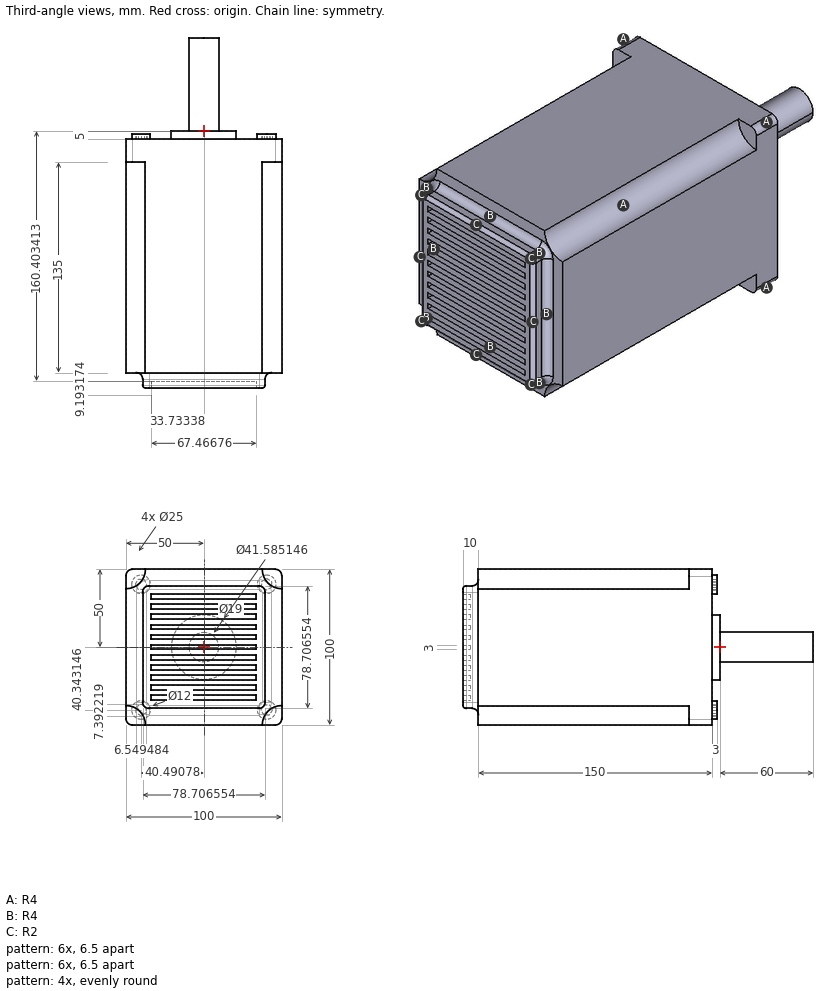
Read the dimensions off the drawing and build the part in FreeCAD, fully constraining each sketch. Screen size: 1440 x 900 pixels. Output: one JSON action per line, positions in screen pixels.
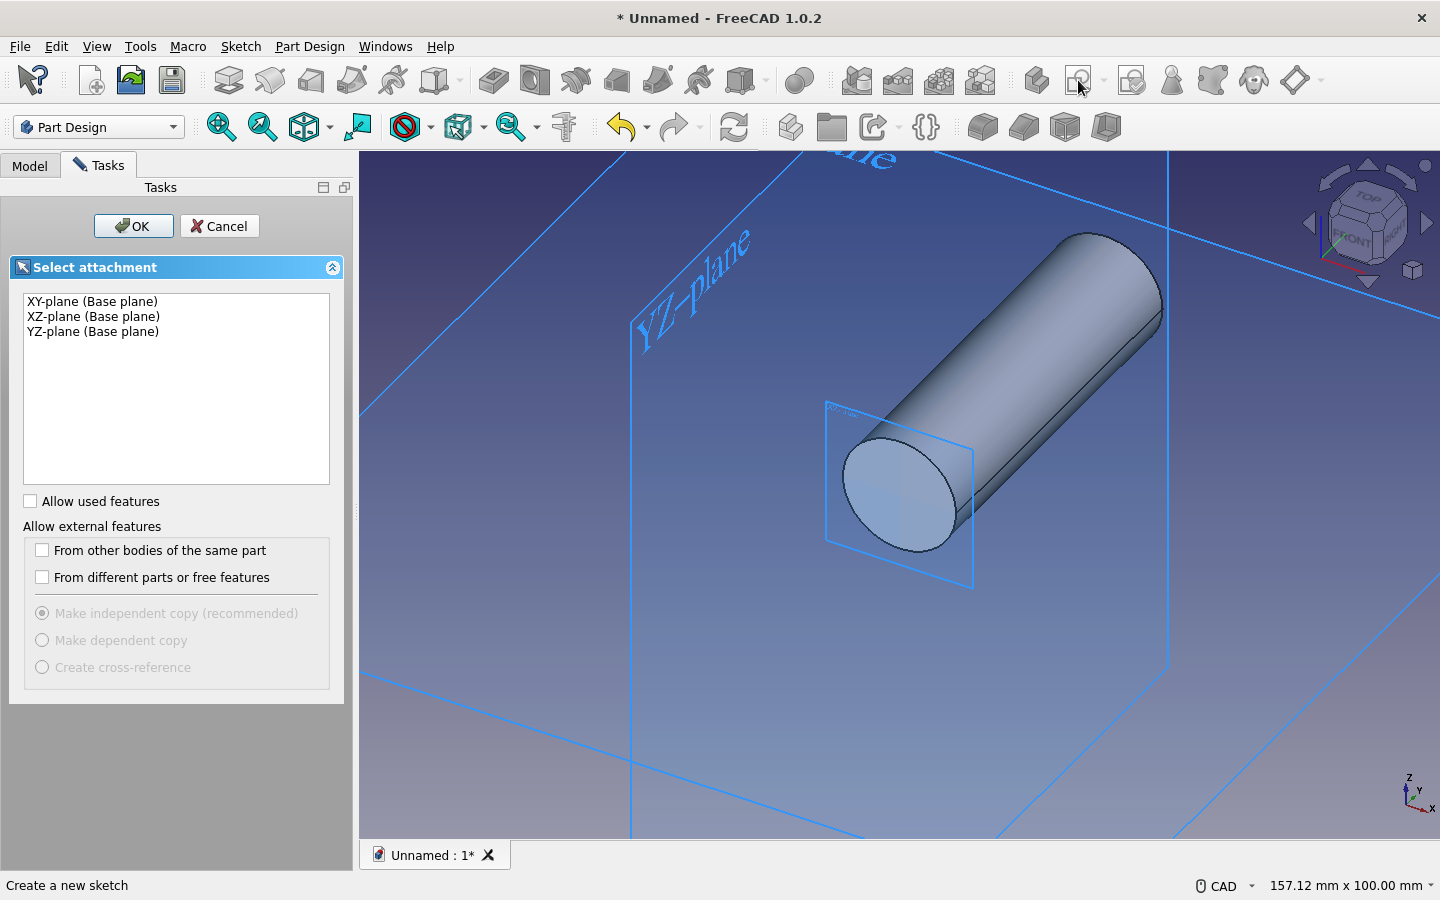
{"action": "left_click", "coordinate": [84, 316]}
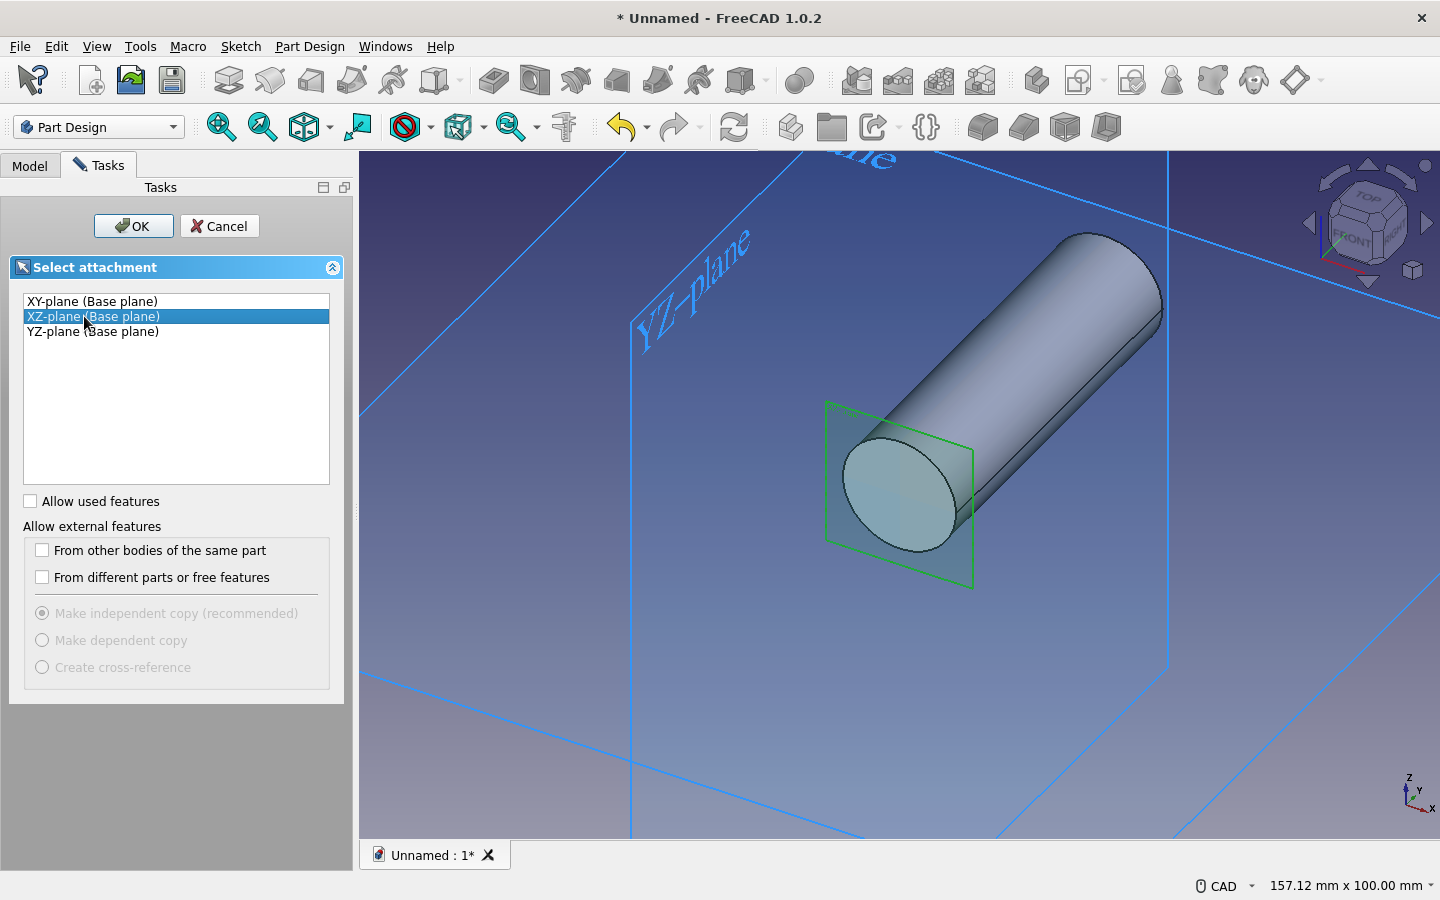
{"action": "left_click", "coordinate": [134, 226]}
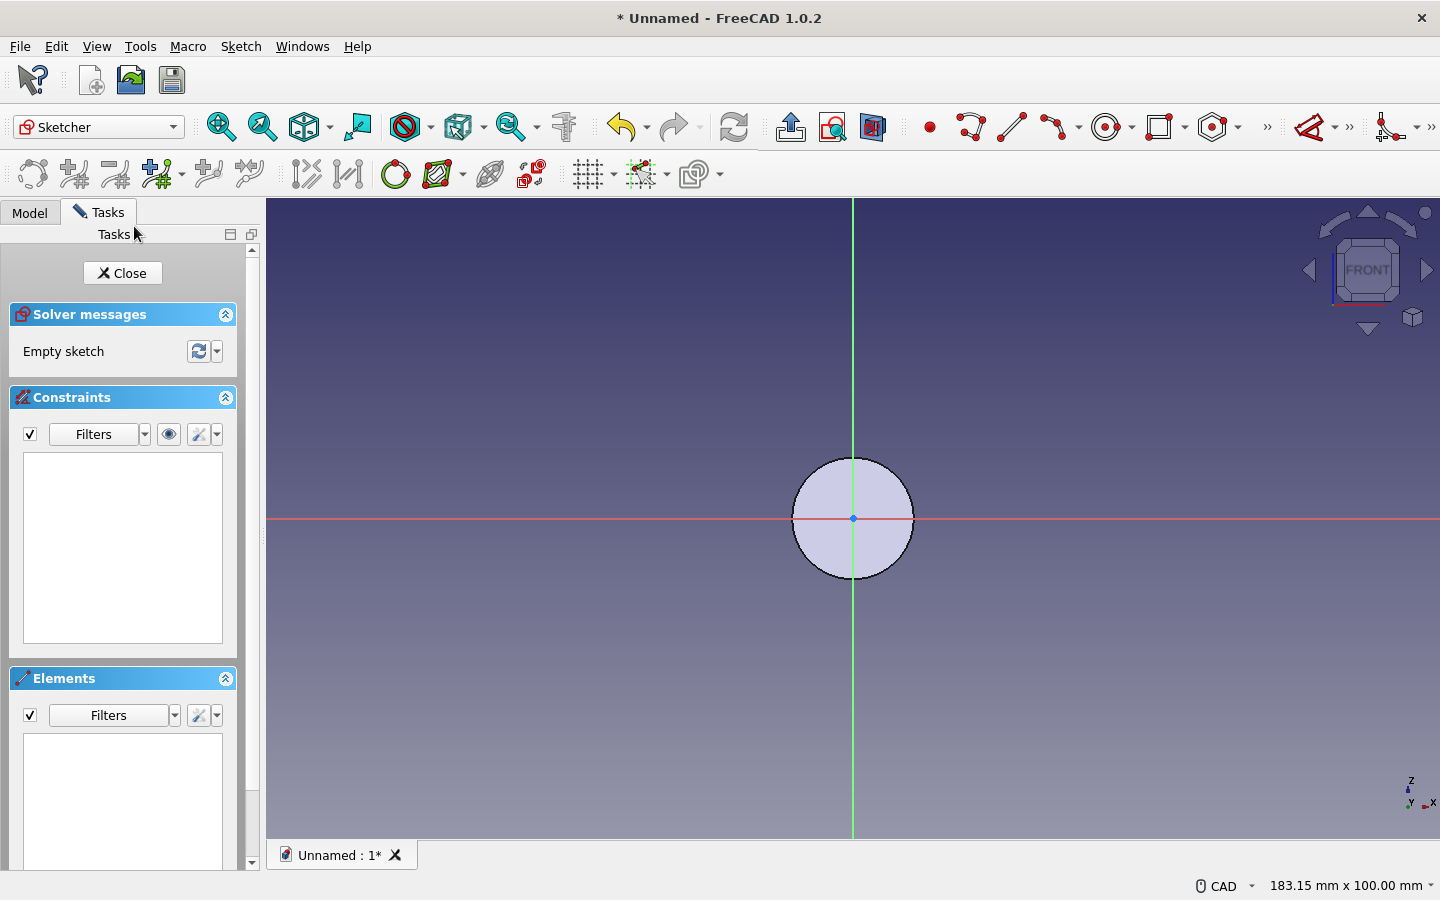
{"action": "scroll", "coordinate": [992, 519], "scroll_direction": "up", "scroll_amount": 2}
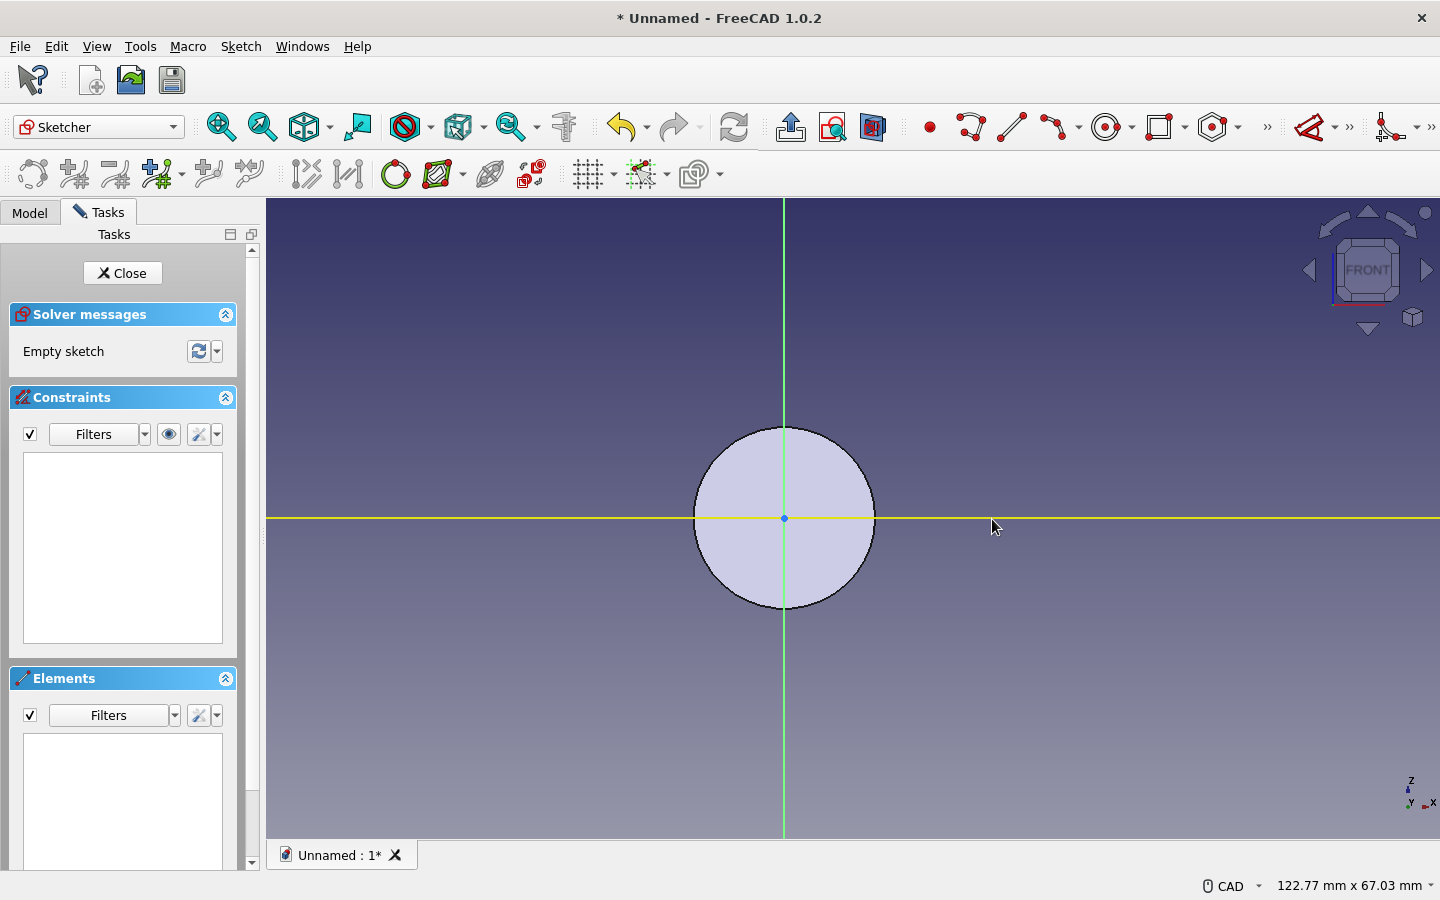
{"action": "left_click", "coordinate": [1106, 128]}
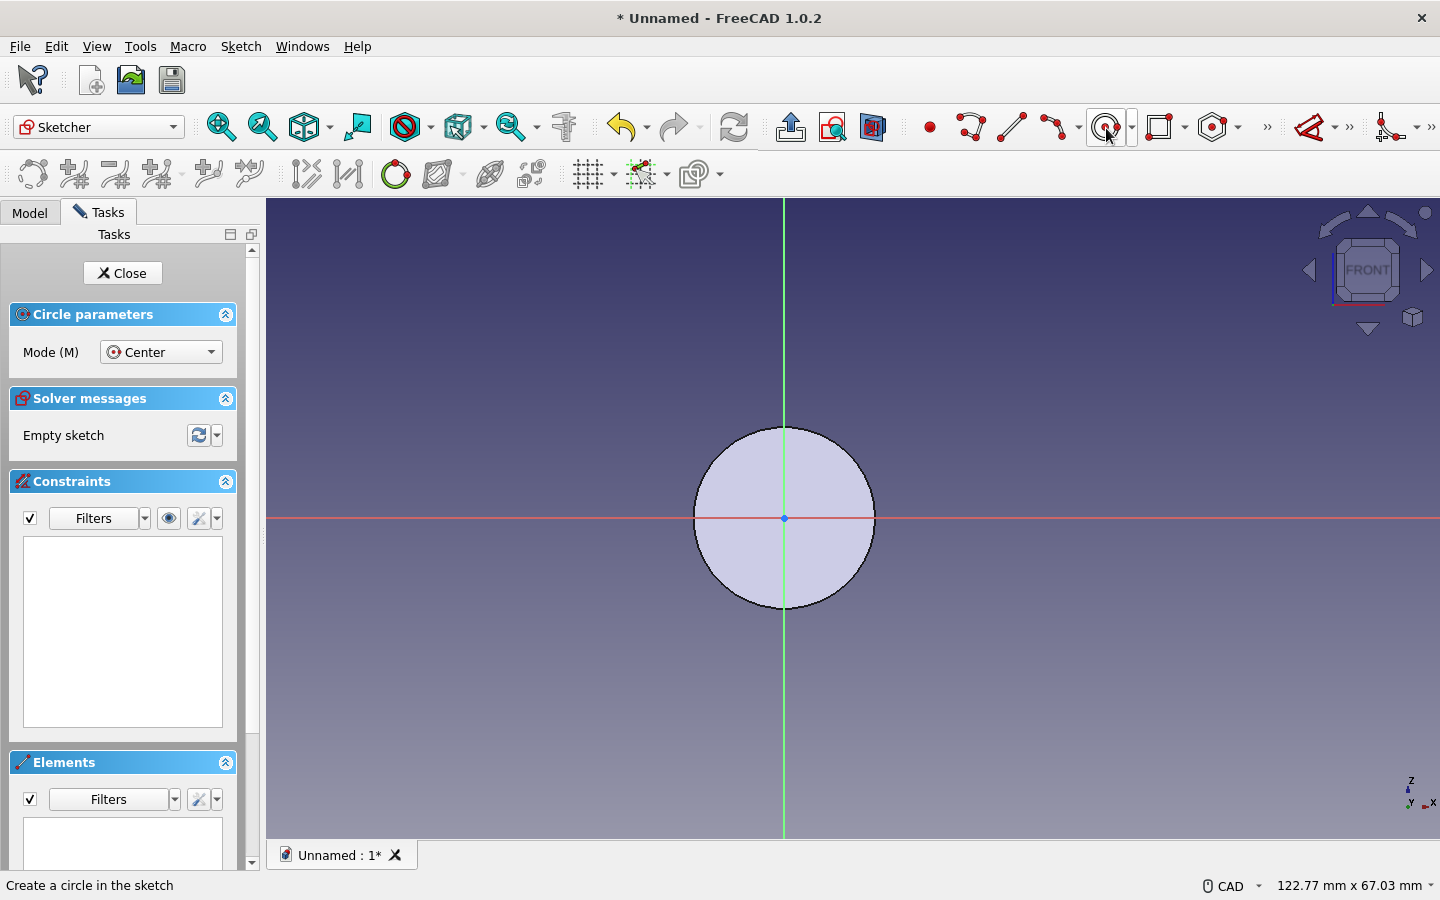
{"action": "left_click", "coordinate": [784, 518]}
{"action": "left_click", "coordinate": [925, 377]}
{"action": "key", "text": "Escape"}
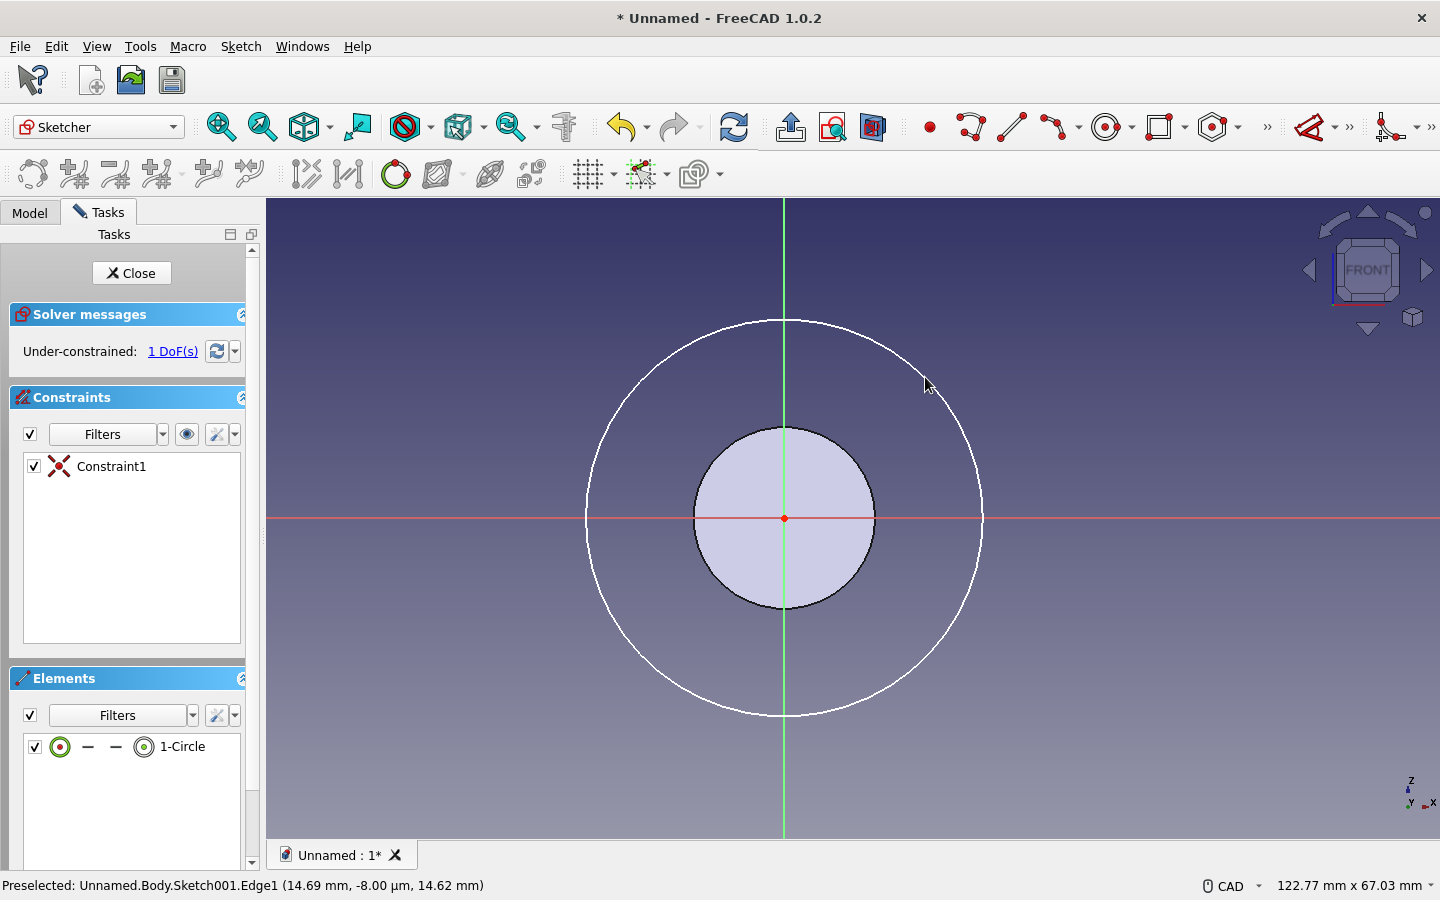
{"action": "left_click", "coordinate": [1308, 128]}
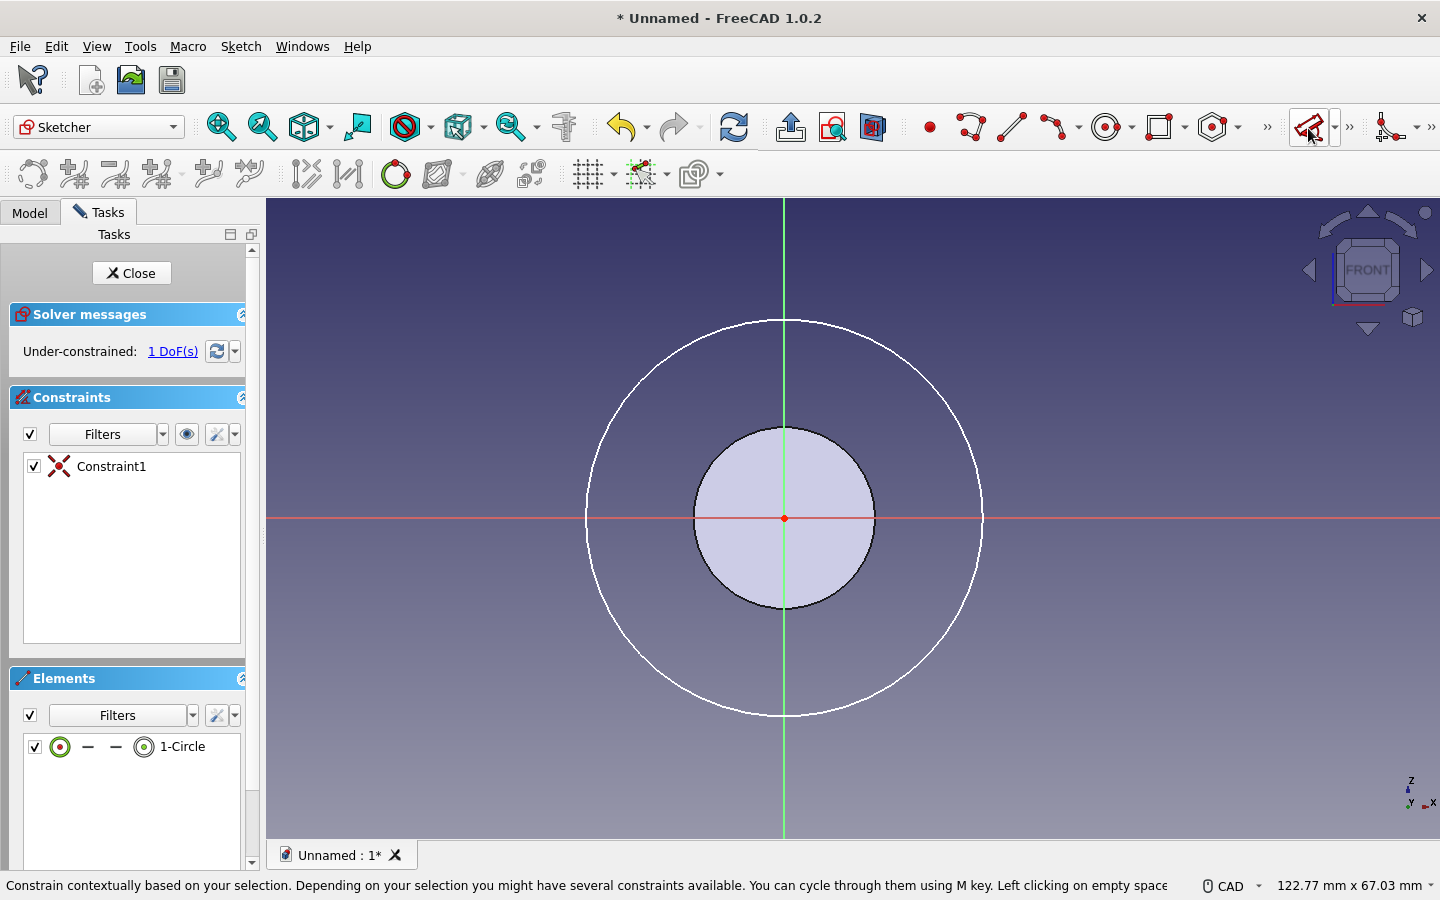
{"action": "left_click", "coordinate": [924, 377]}
{"action": "left_click", "coordinate": [947, 354]}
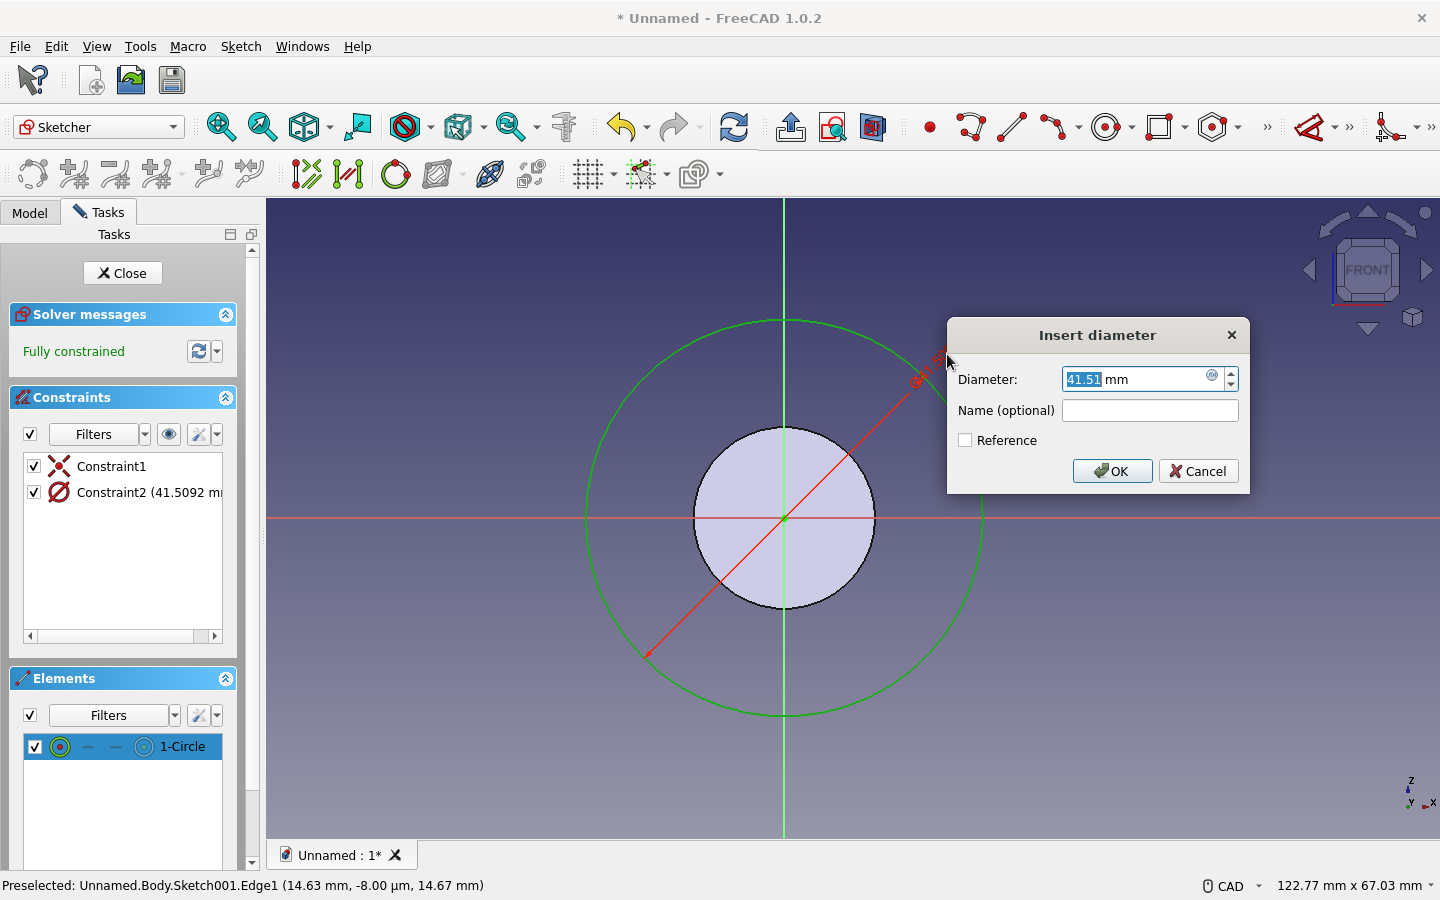
{"action": "type", "text": "41.585146"}
{"action": "key", "text": "Return"}
{"action": "key", "text": "Escape"}